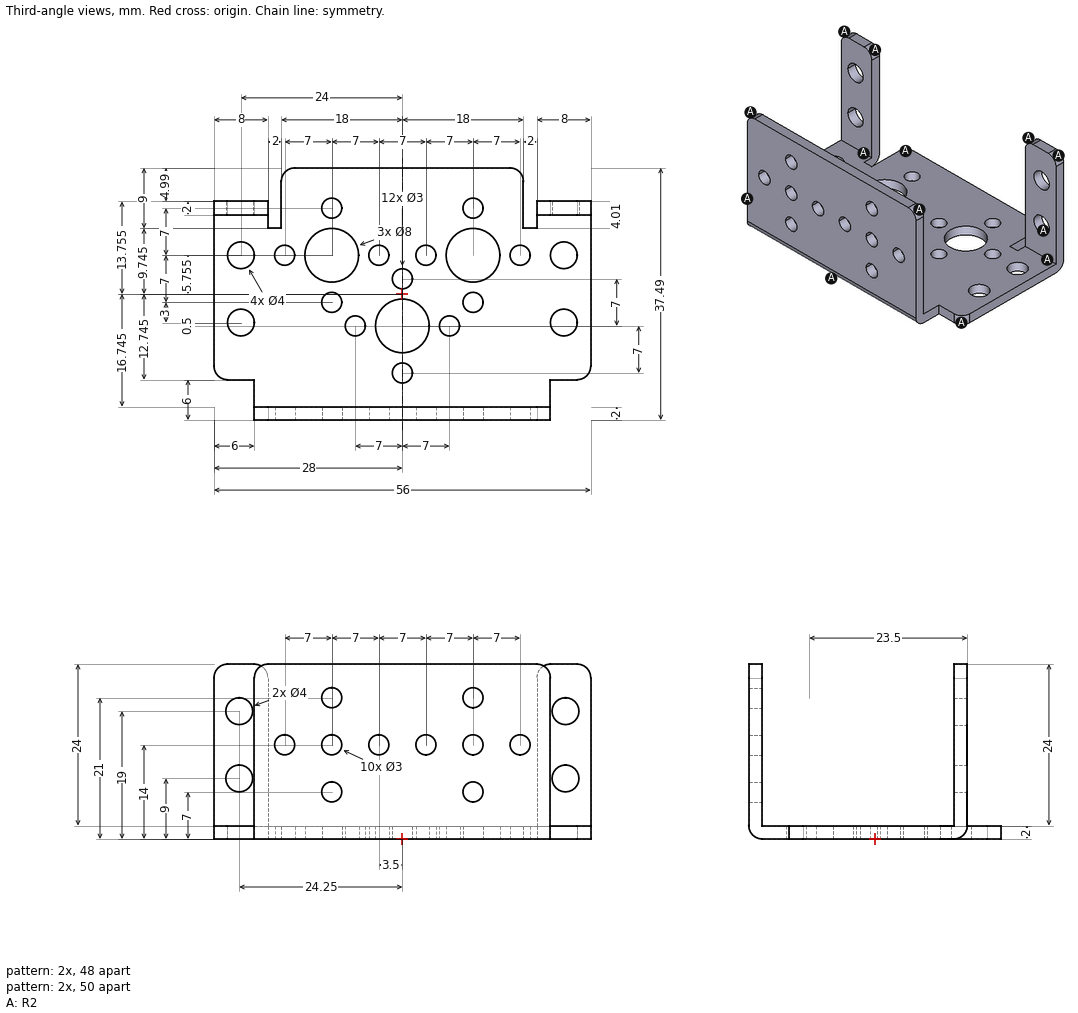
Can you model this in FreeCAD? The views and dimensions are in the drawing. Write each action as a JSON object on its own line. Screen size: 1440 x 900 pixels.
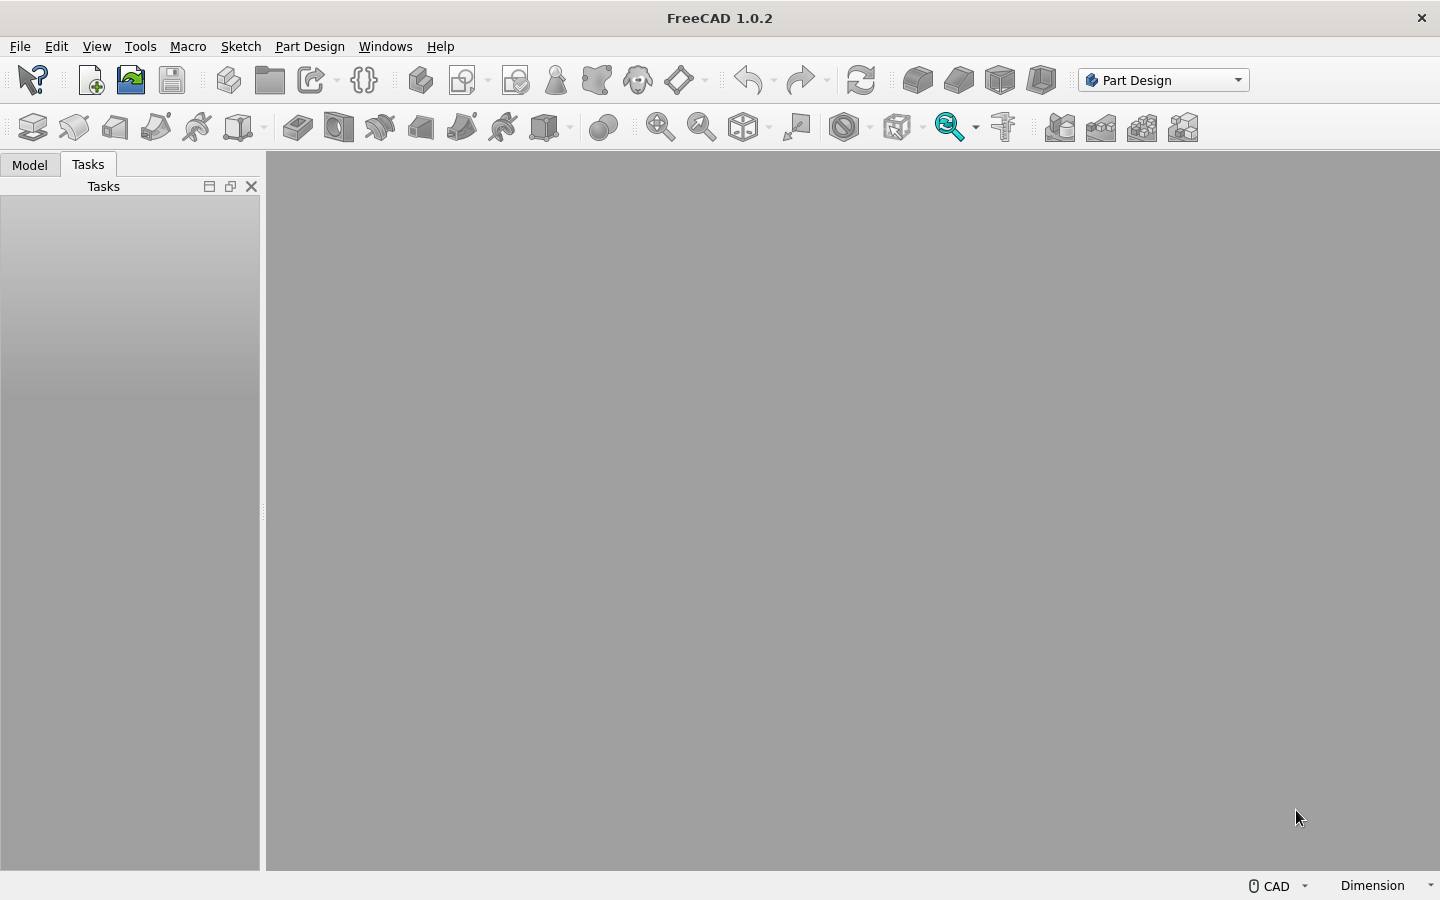
{"action": "key", "text": "ctrl+n"}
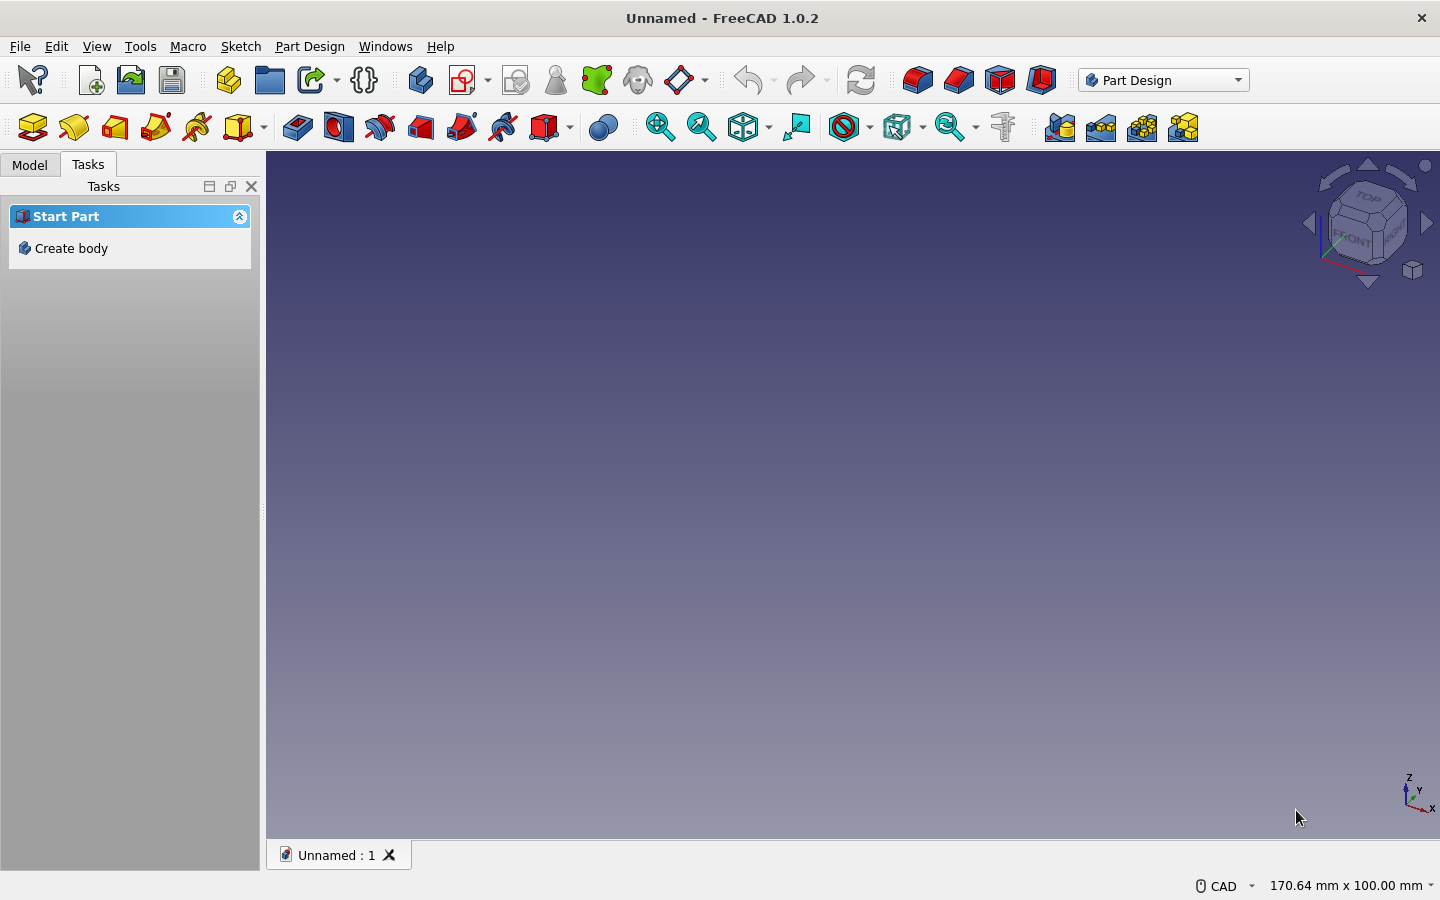
{"action": "left_click", "coordinate": [462, 80]}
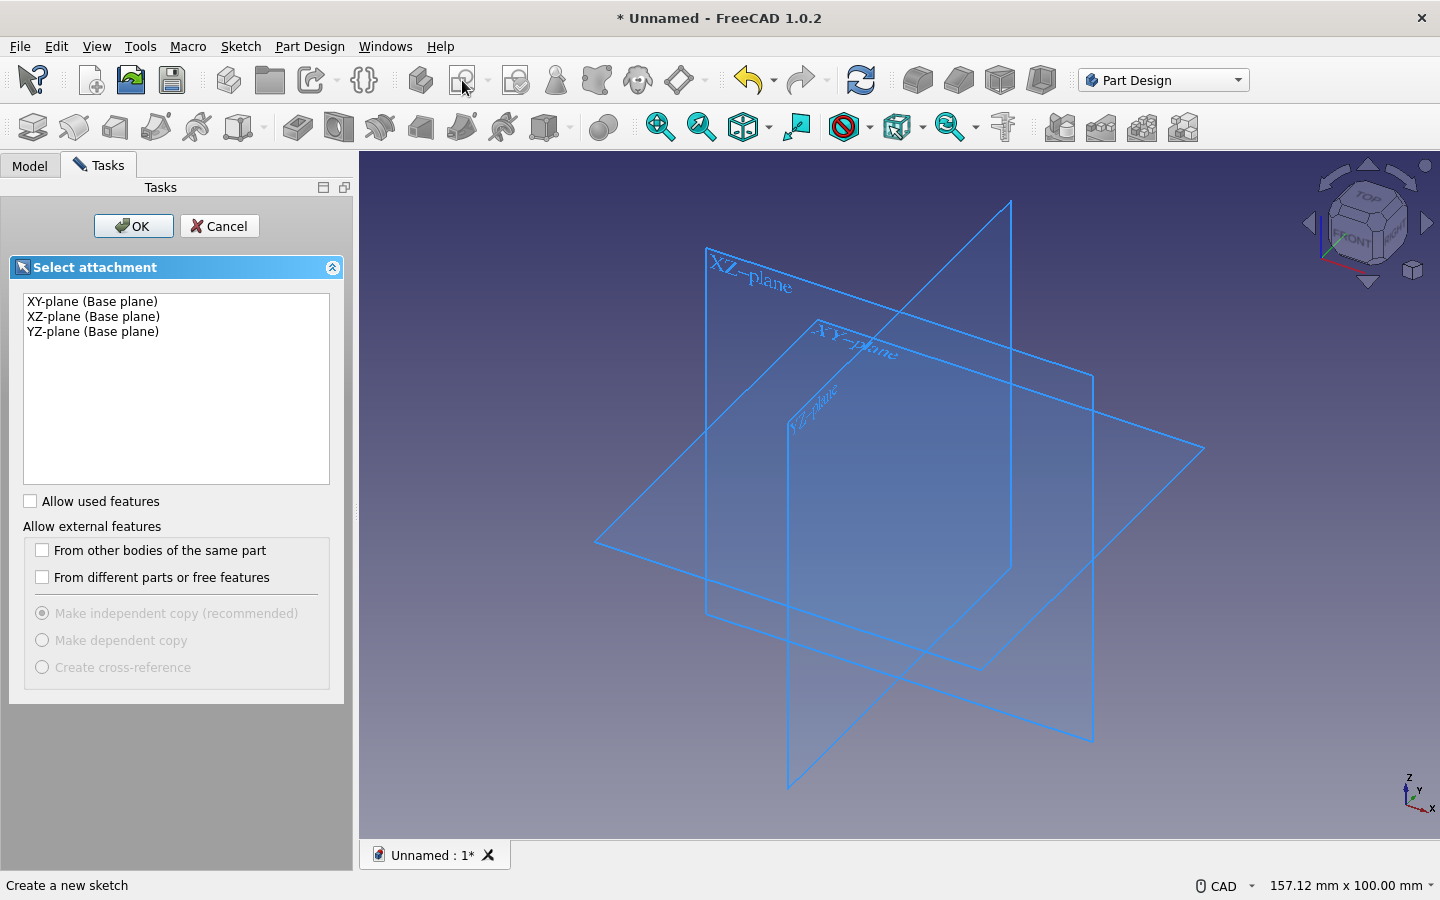
{"action": "left_click", "coordinate": [84, 302]}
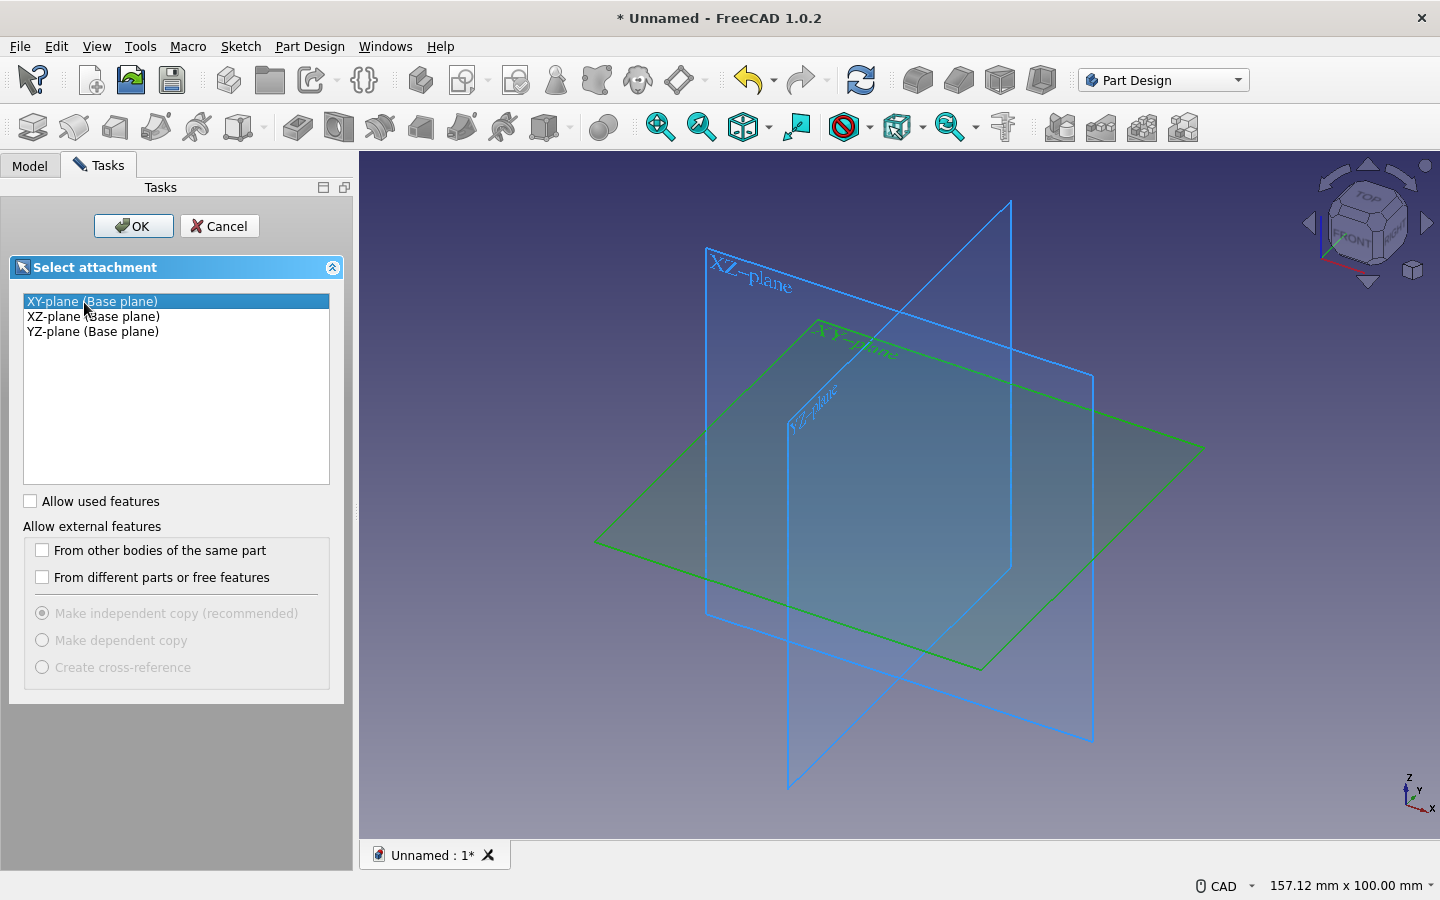
{"action": "left_click", "coordinate": [134, 226]}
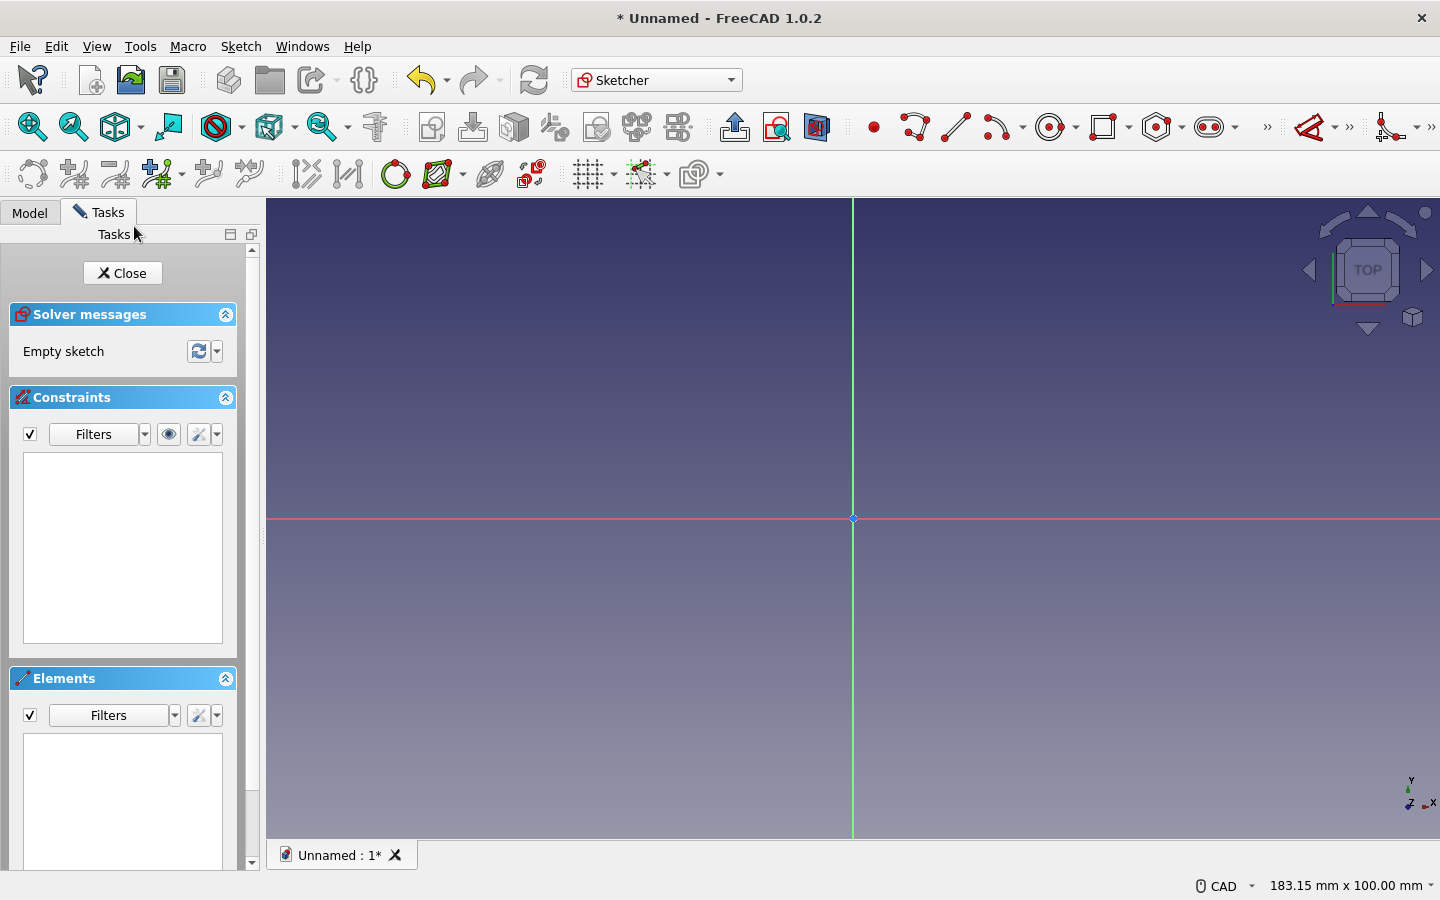
{"action": "scroll", "coordinate": [936, 518], "scroll_direction": "up", "scroll_amount": 3}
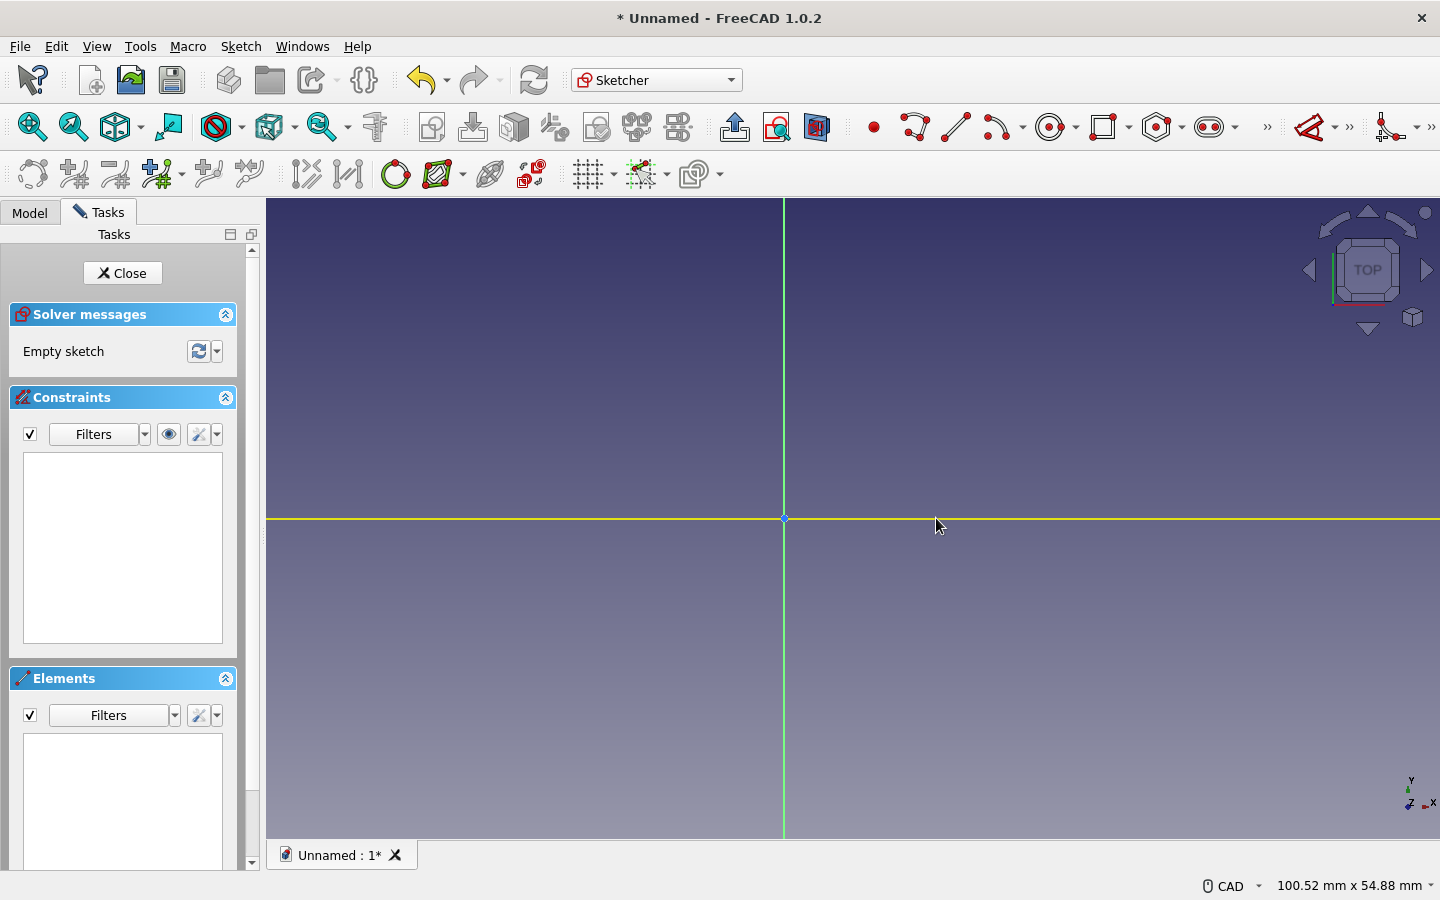
{"action": "key", "text": "g v"}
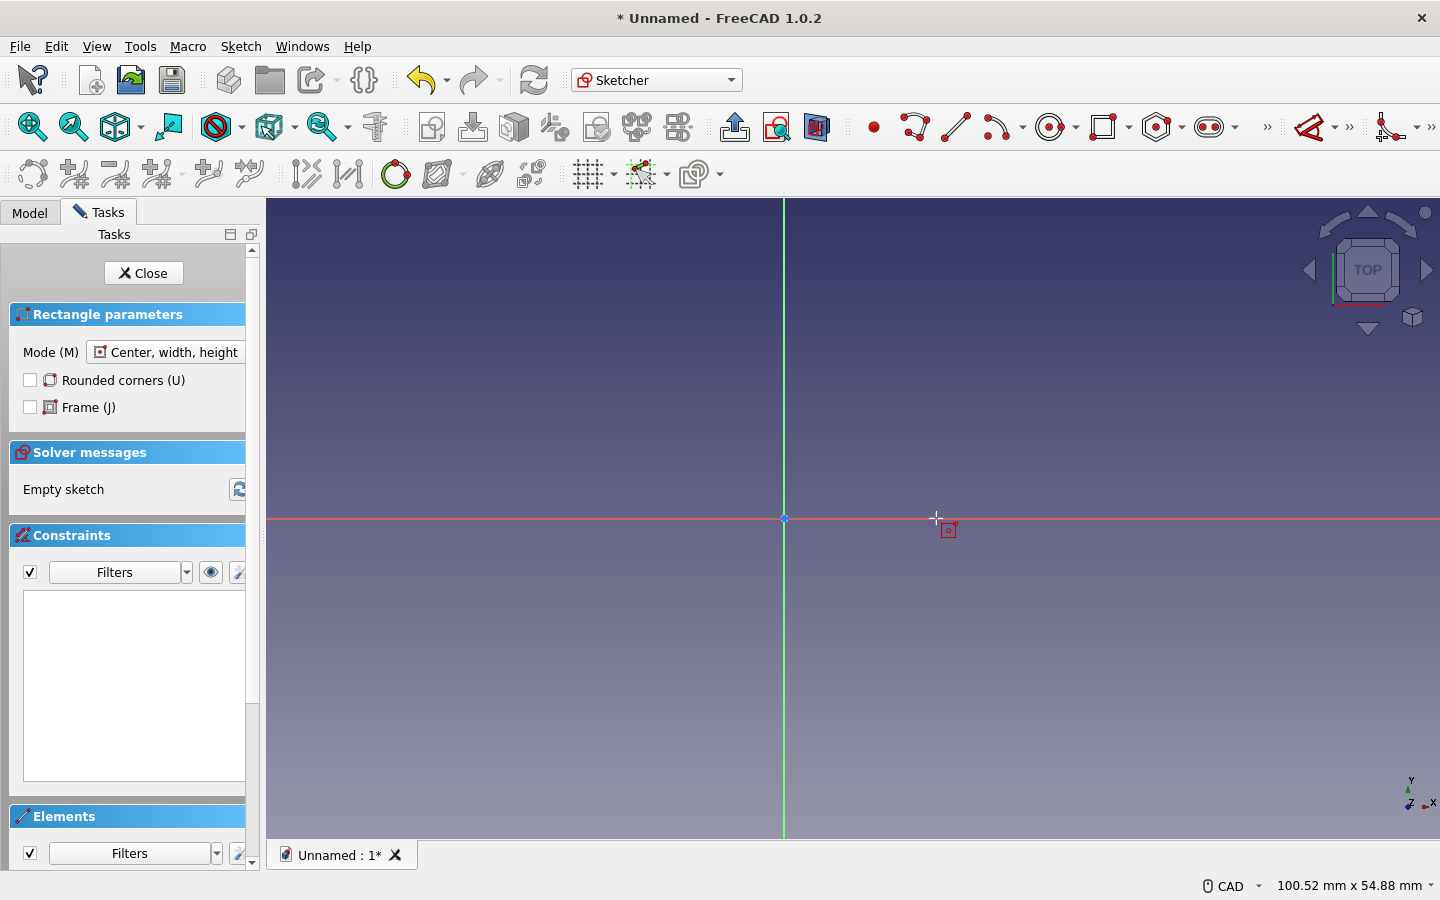
{"action": "left_click", "coordinate": [784, 518]}
{"action": "mouse_move", "coordinate": [1111, 300]}